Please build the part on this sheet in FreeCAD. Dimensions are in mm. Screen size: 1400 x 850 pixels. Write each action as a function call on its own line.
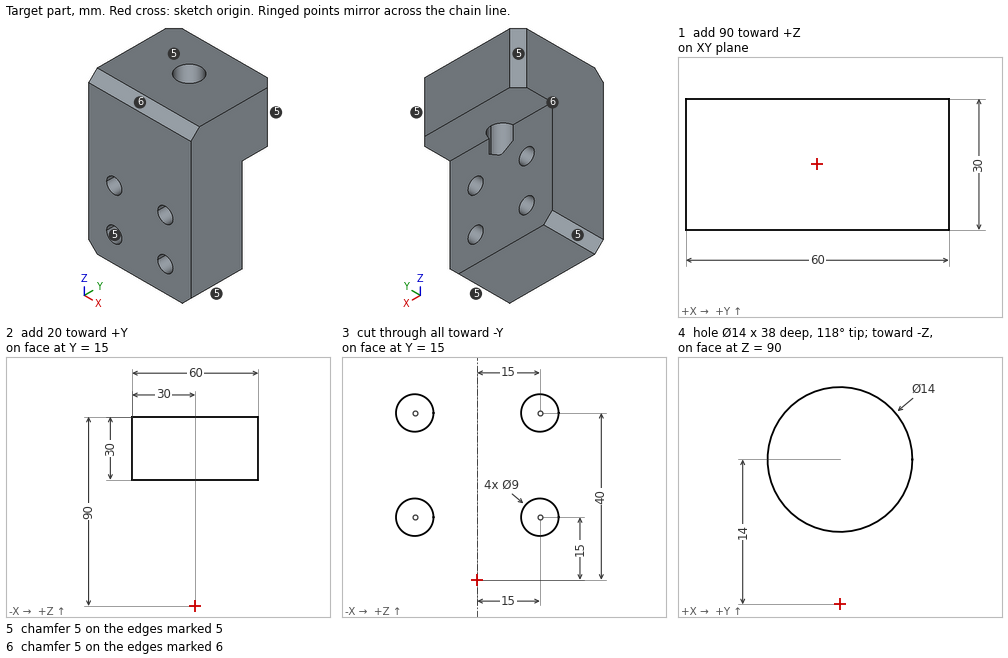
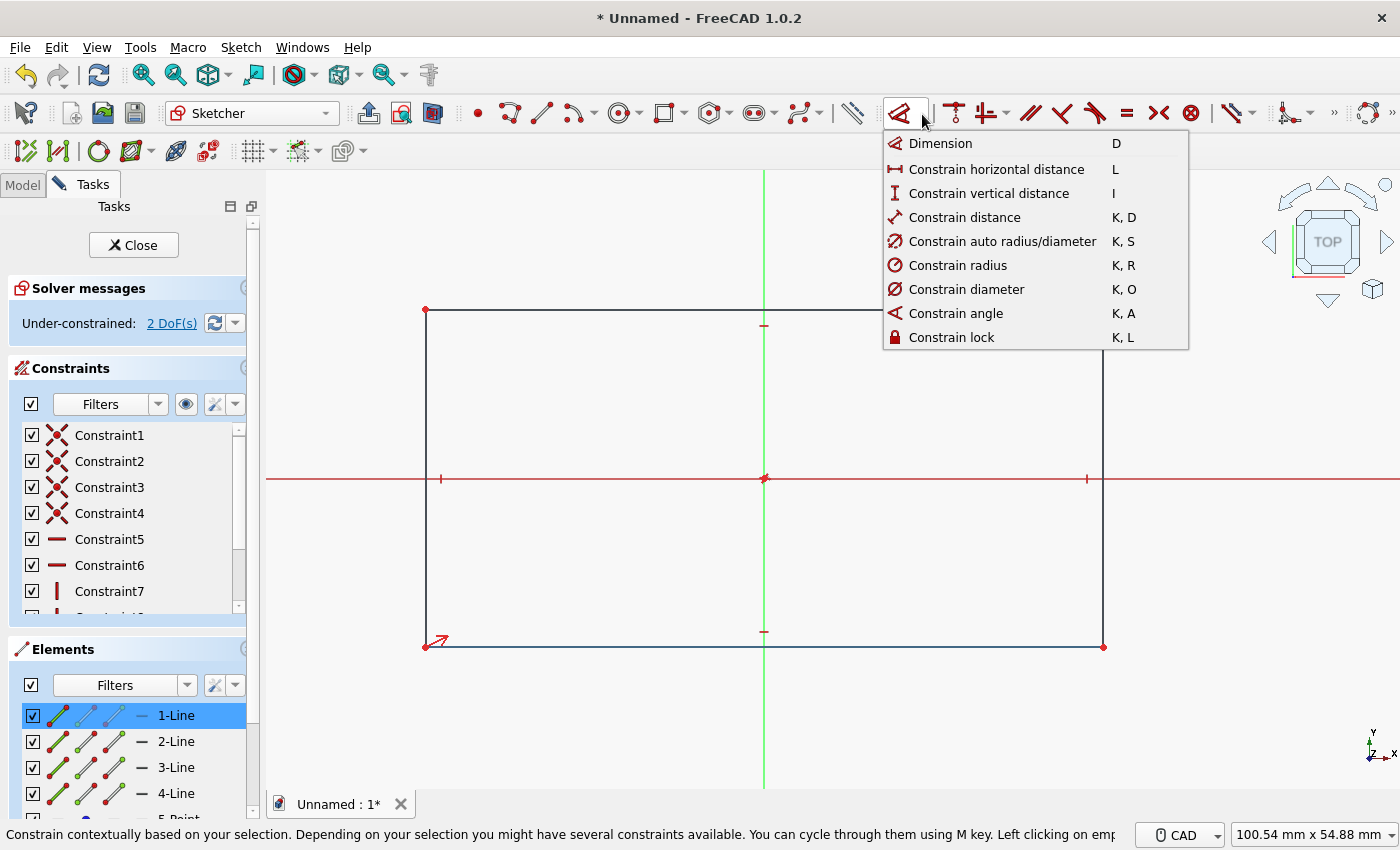
click(1036, 169)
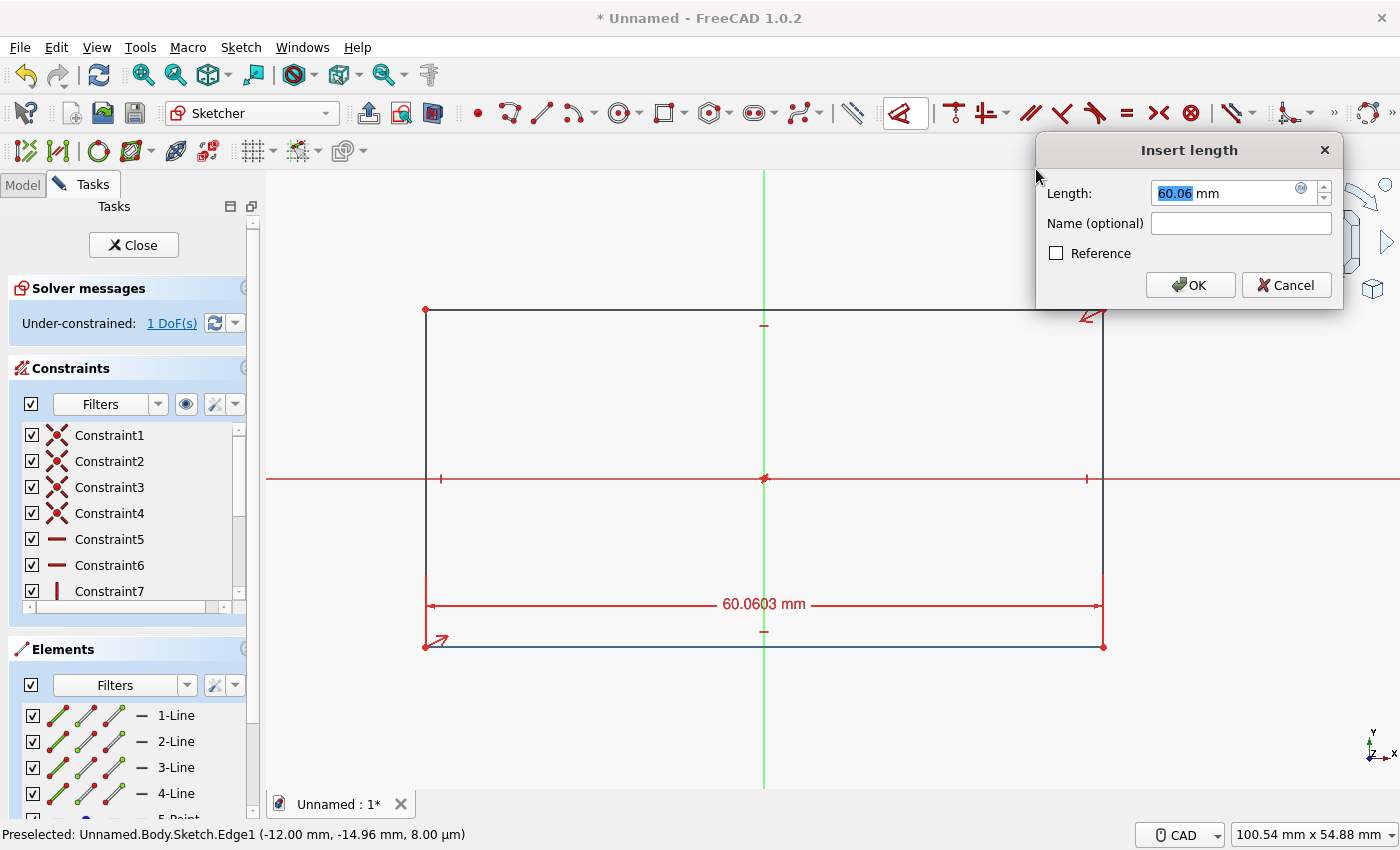
text(60)
key(Return)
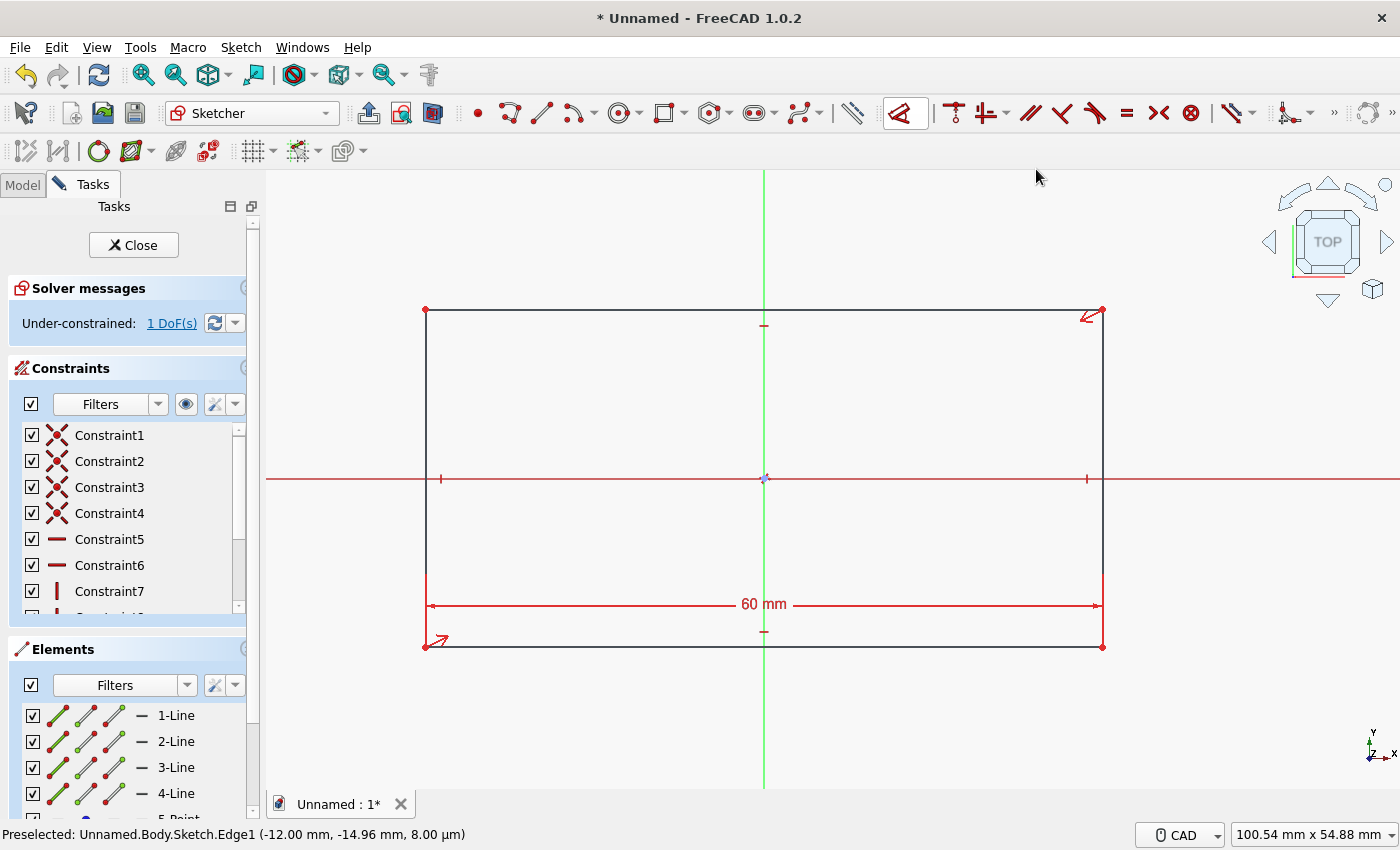
click(1103, 546)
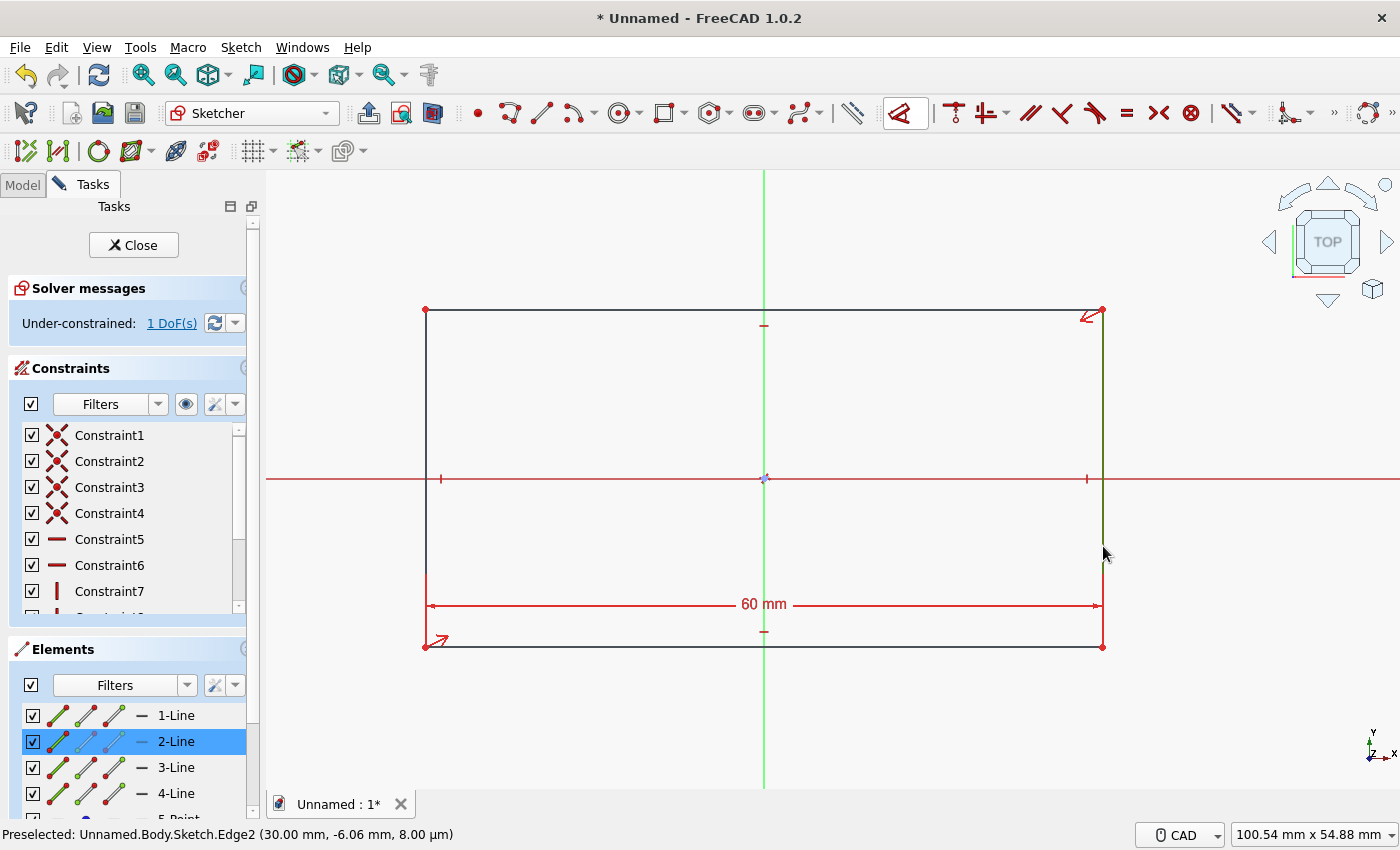
key(i)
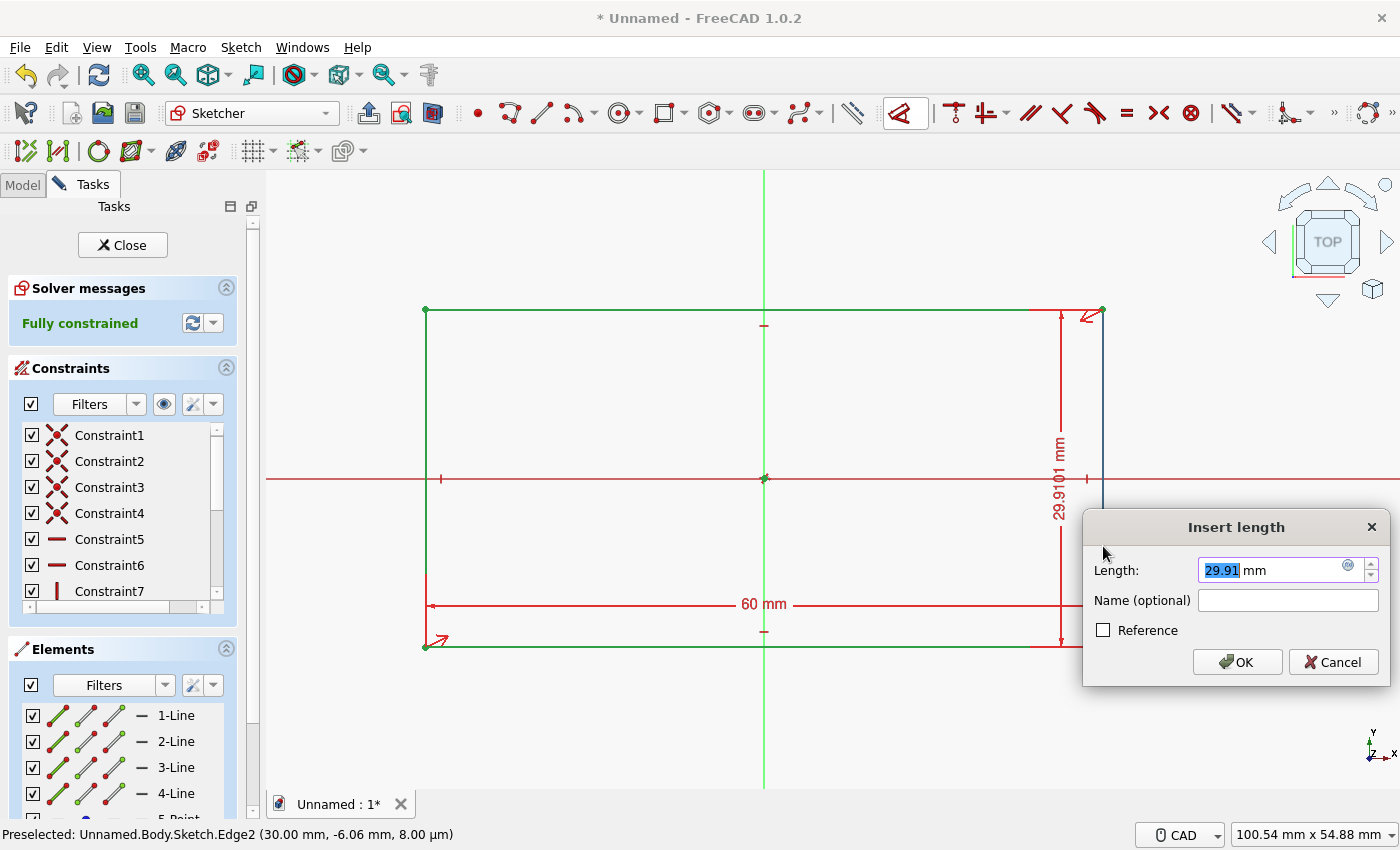
text(30)
key(Return)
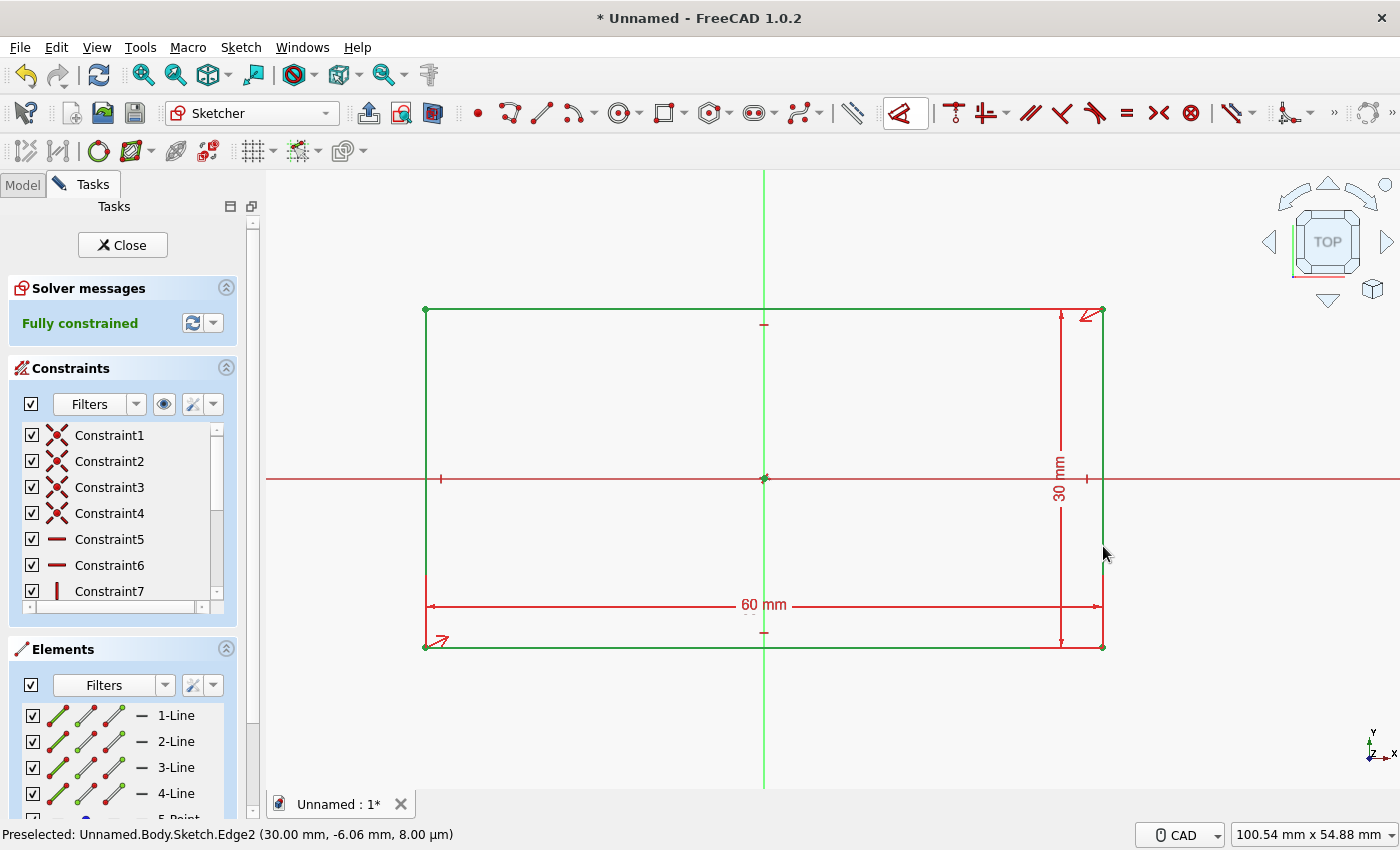
click(123, 245)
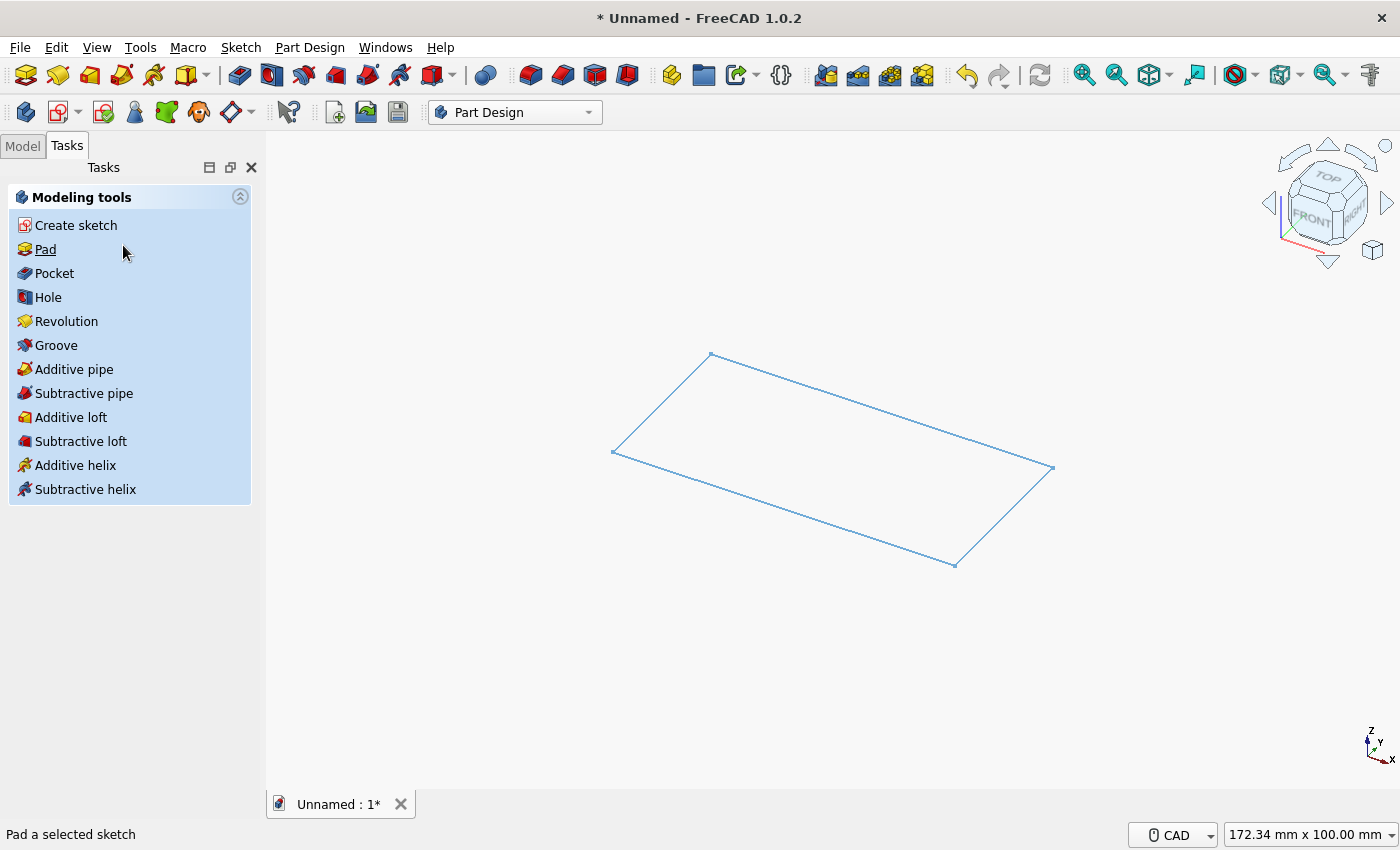
click(26, 76)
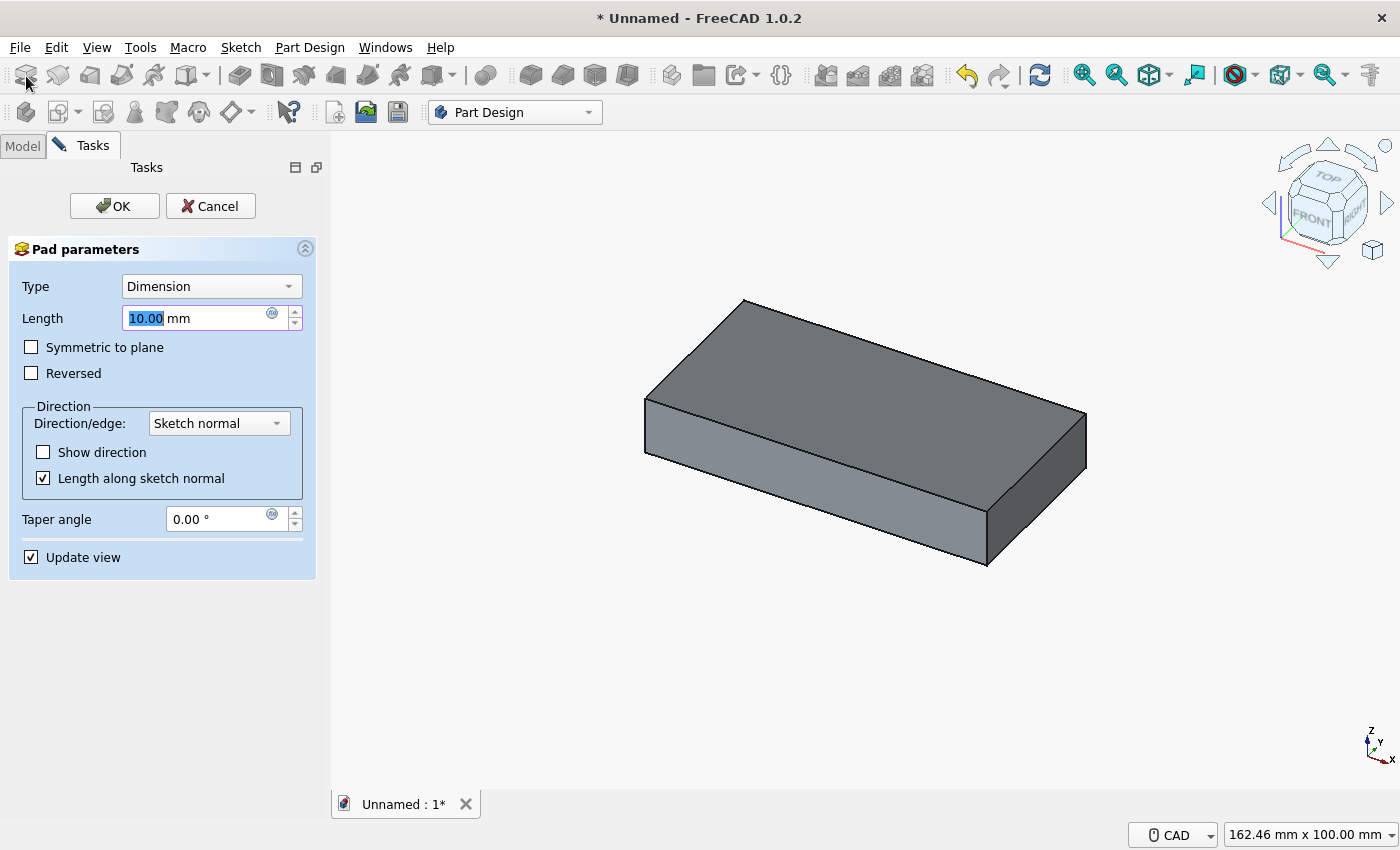
text(90)
key(Tab)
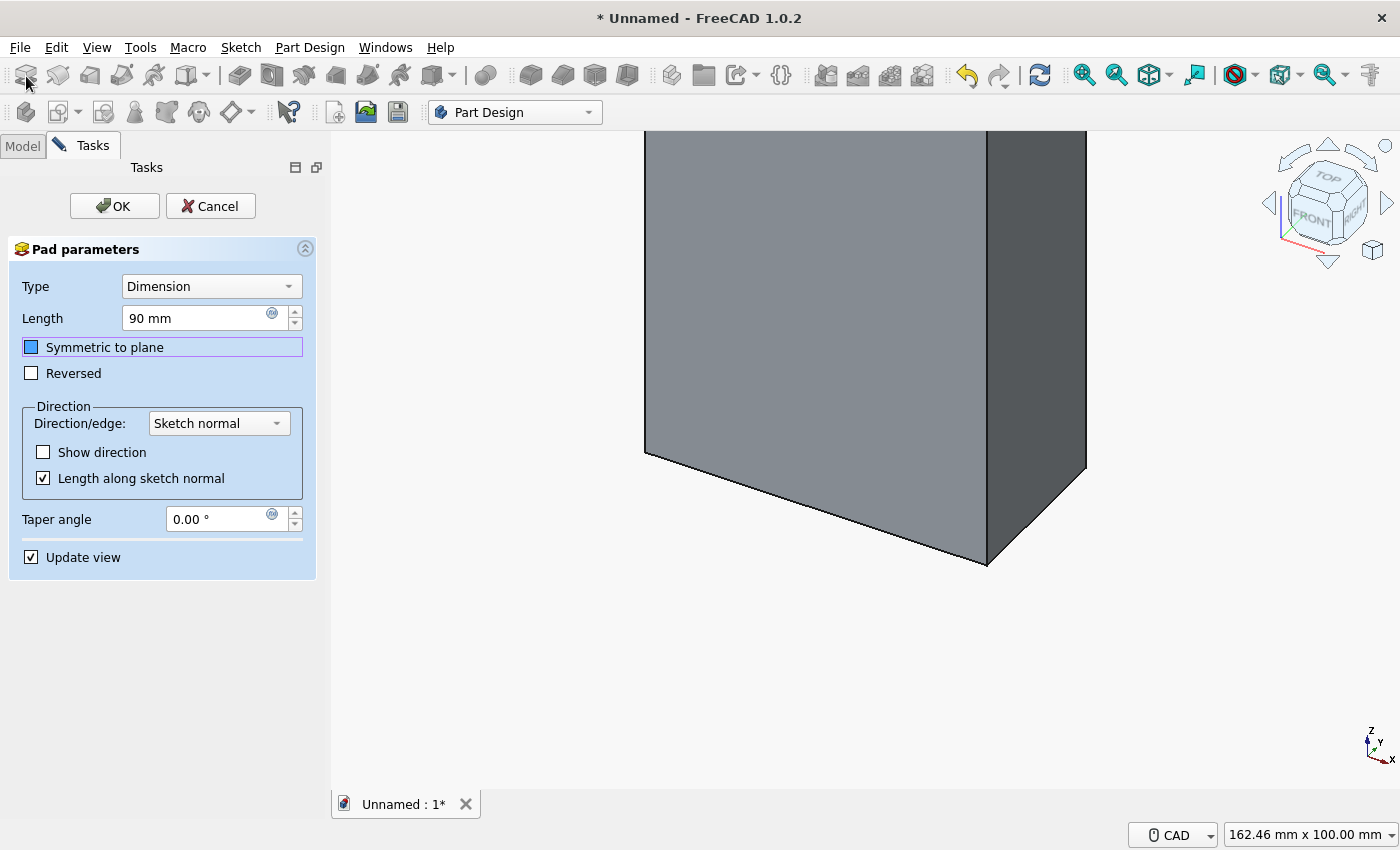
click(115, 206)